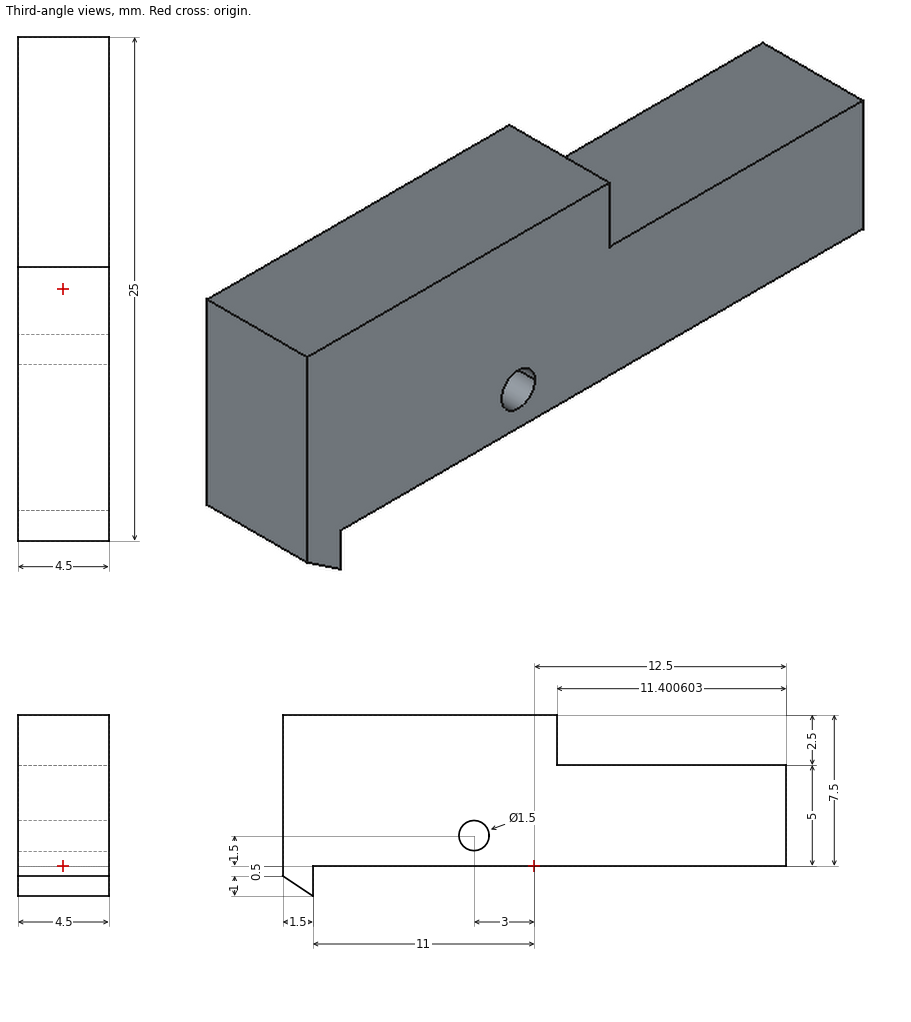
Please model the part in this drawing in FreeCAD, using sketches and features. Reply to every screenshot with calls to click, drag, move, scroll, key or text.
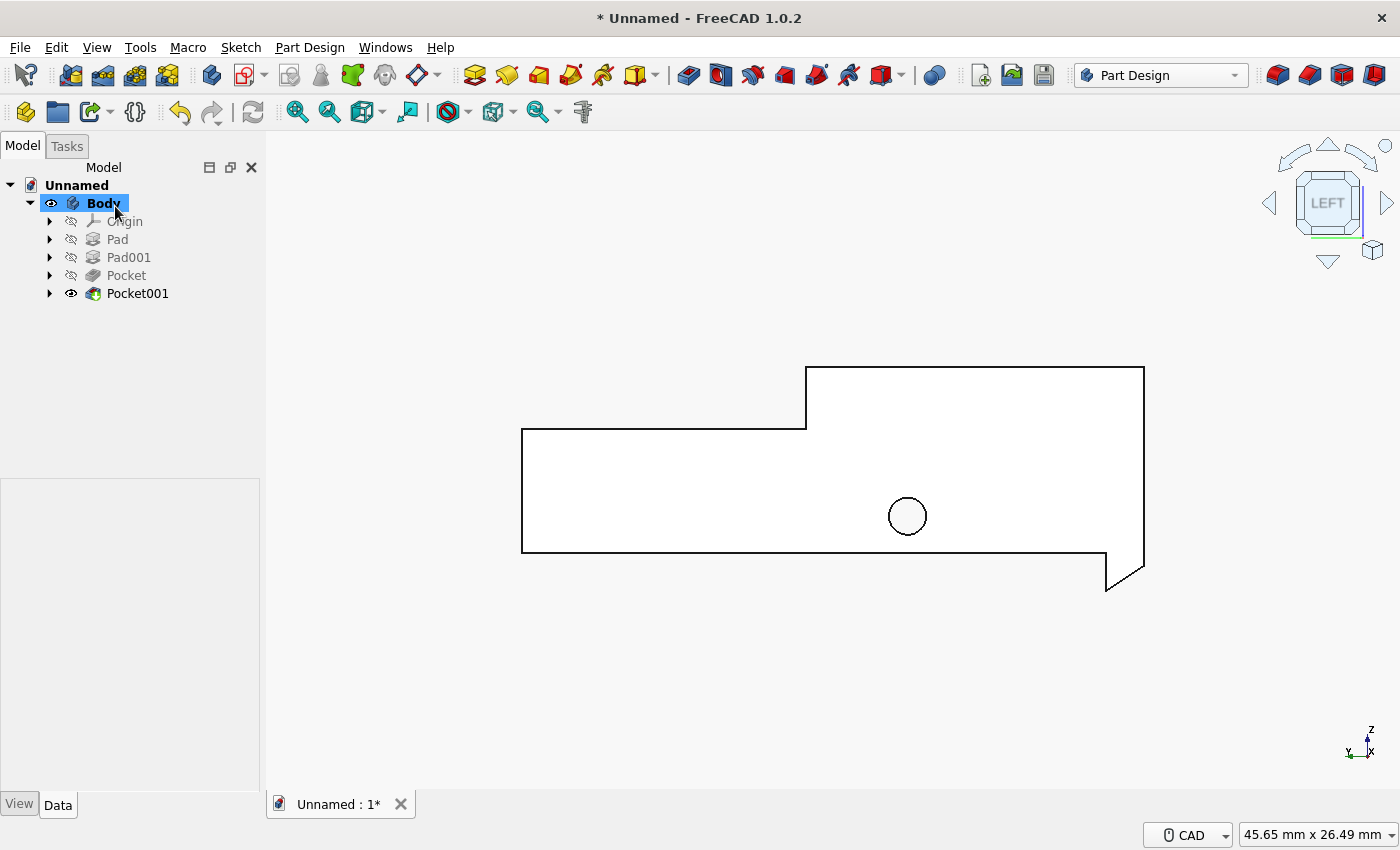
key(0)